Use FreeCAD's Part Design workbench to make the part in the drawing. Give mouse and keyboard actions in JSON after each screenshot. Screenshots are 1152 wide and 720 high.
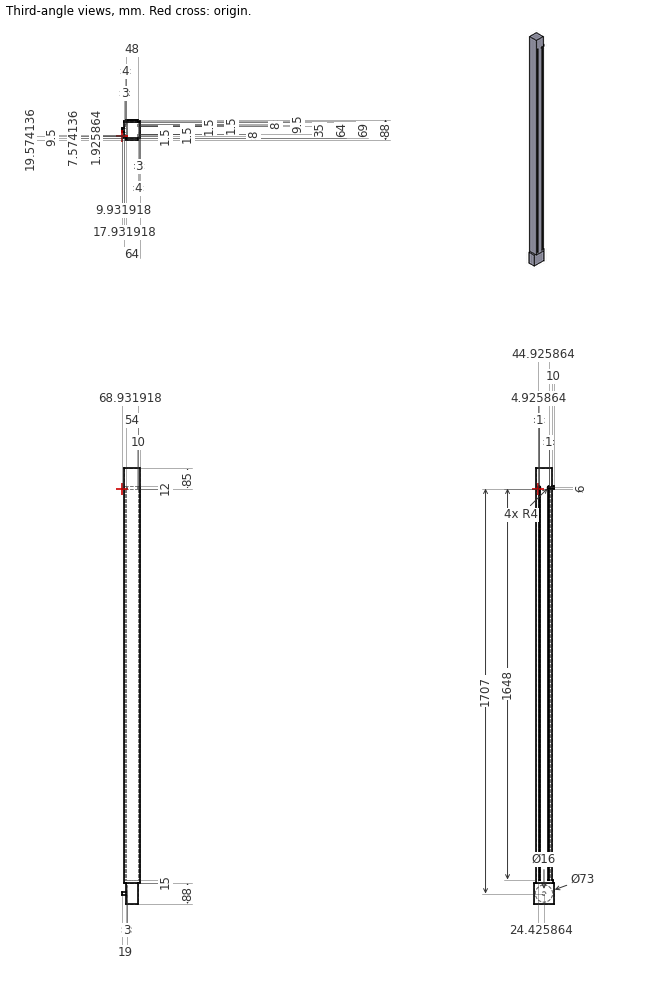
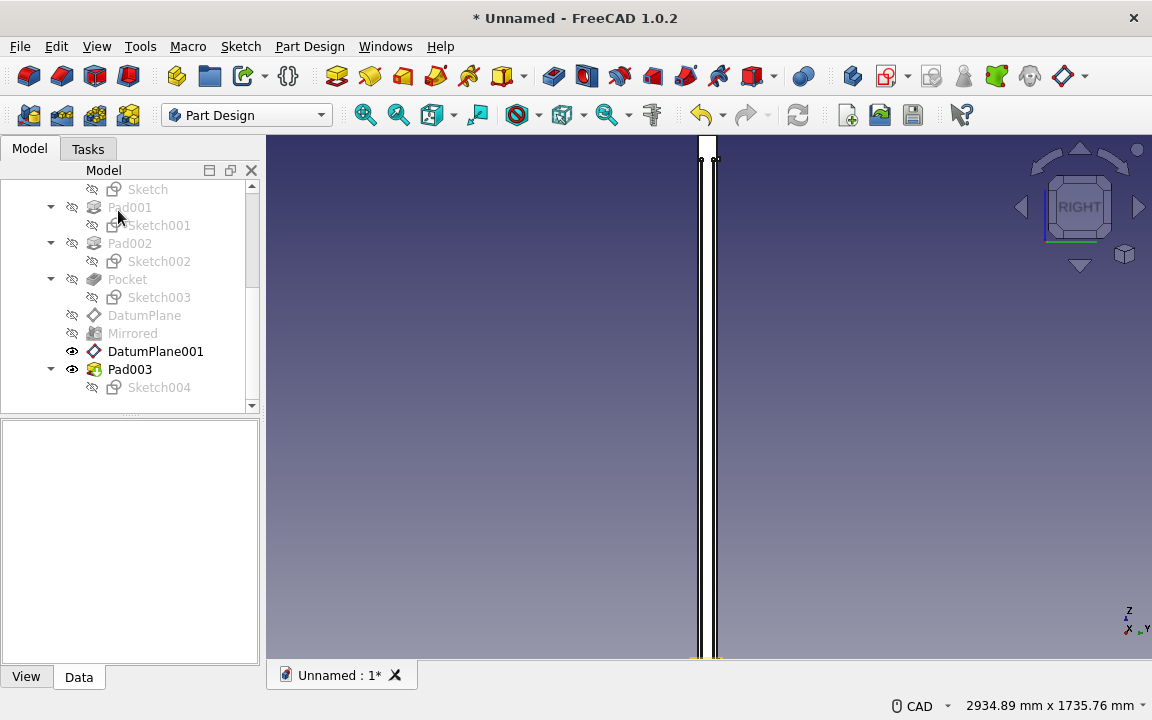
{"action": "left_click", "coordinate": [117, 351]}
{"action": "key", "text": "space"}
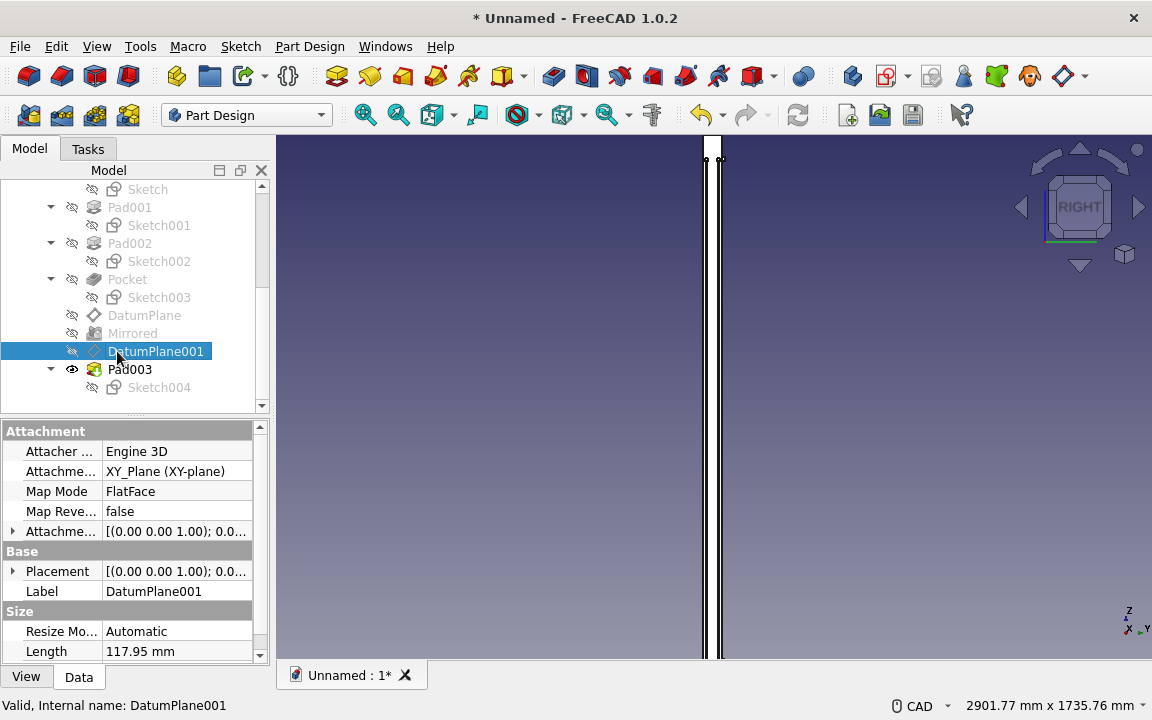
{"action": "left_click", "coordinate": [366, 116]}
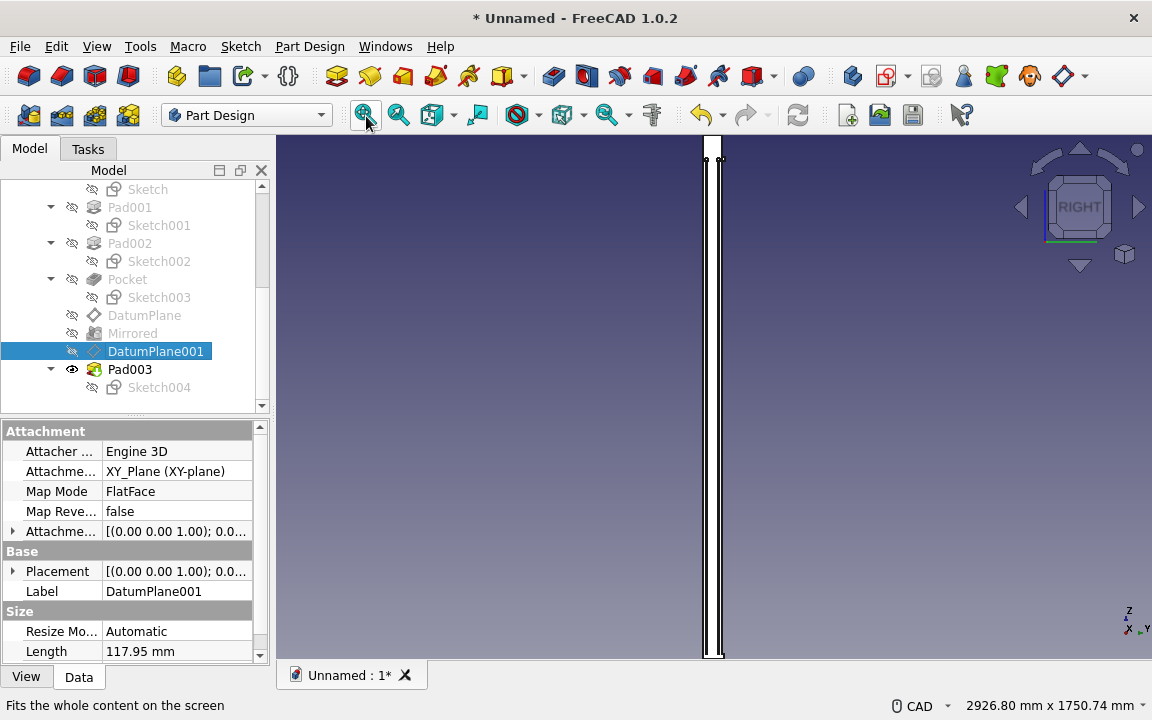
{"action": "key", "text": "5"}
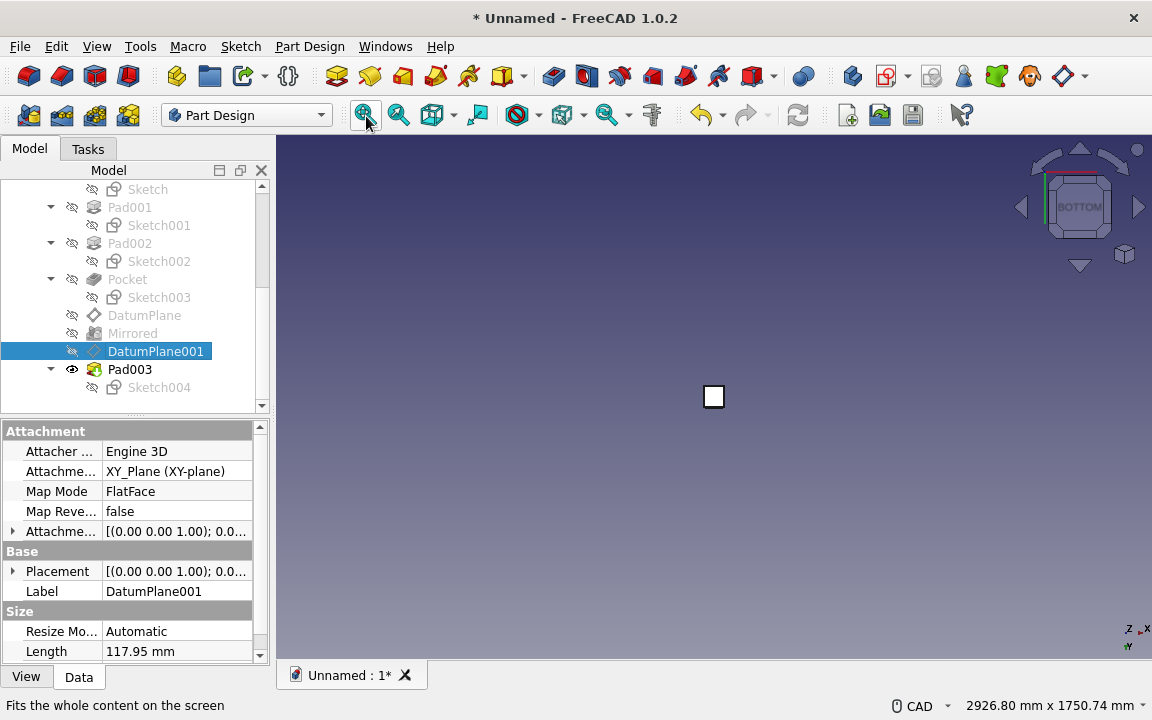
{"action": "left_click", "coordinate": [366, 116]}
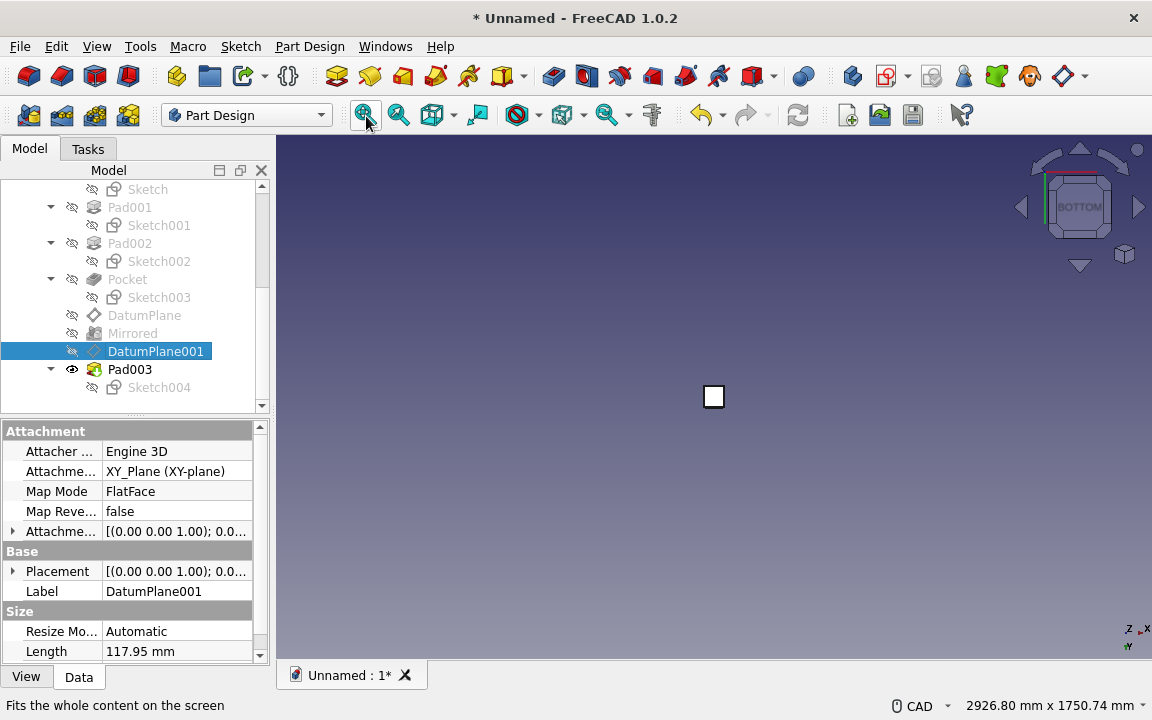
{"action": "left_click", "coordinate": [714, 395]}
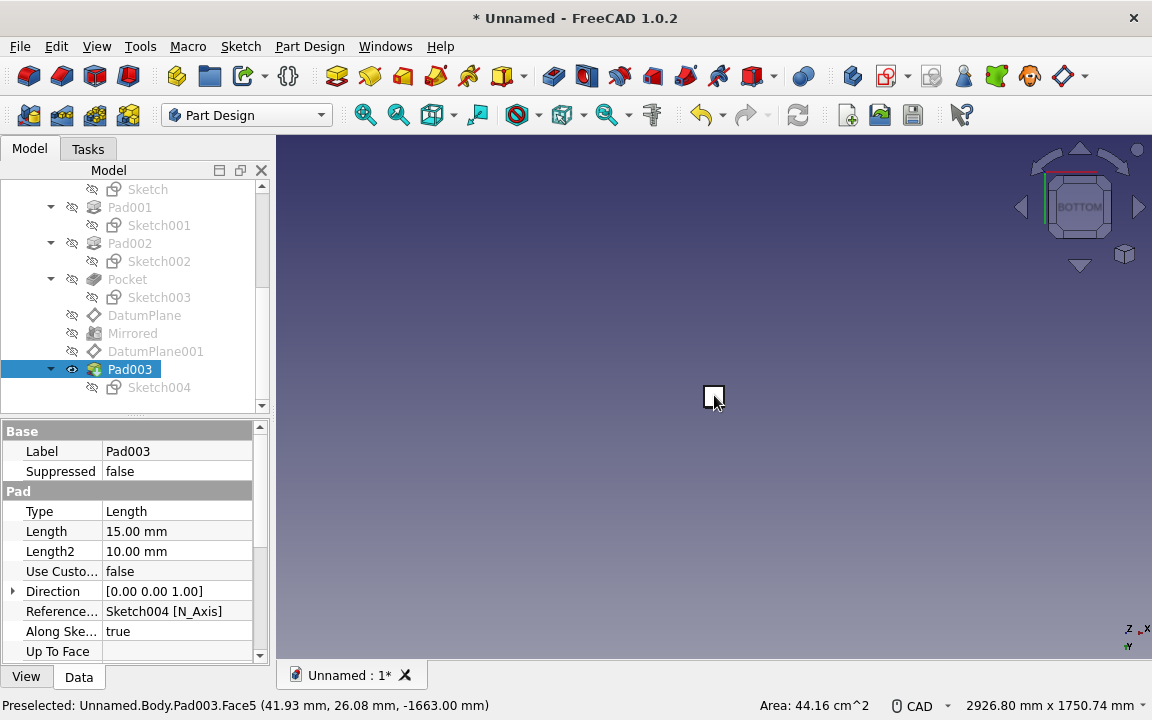
{"action": "left_click", "coordinate": [886, 76]}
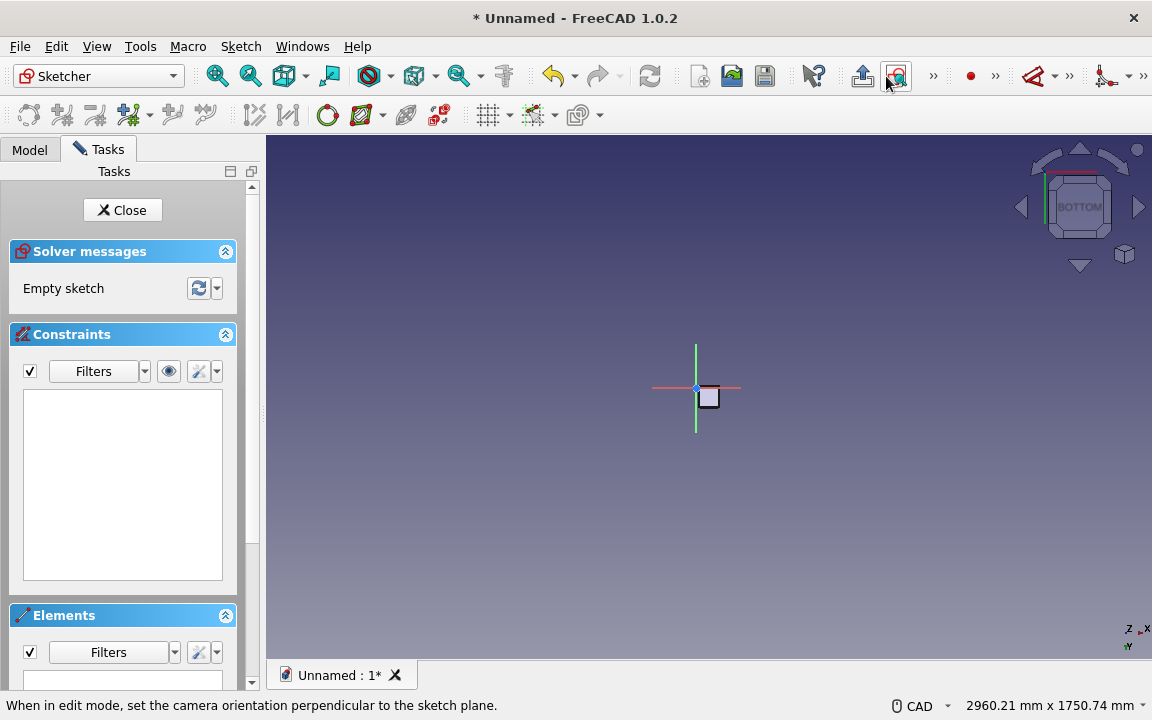
{"action": "scroll", "coordinate": [712, 395], "scroll_direction": "up", "scroll_amount": 13}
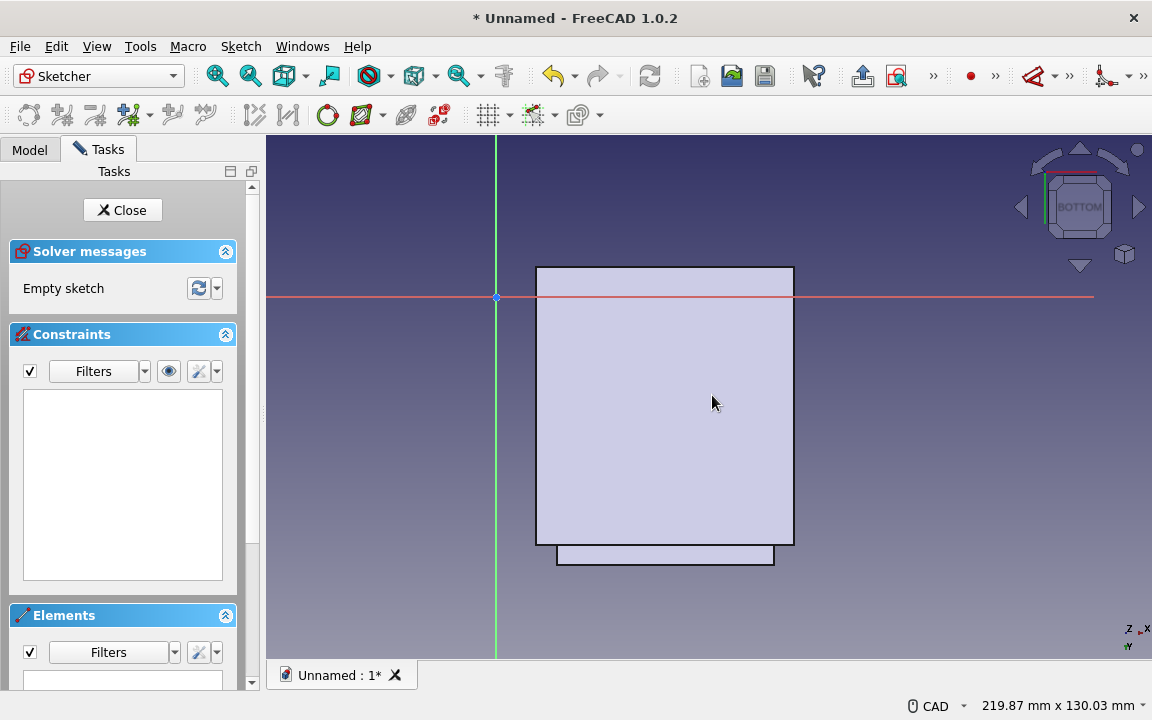
{"action": "key", "text": "g r"}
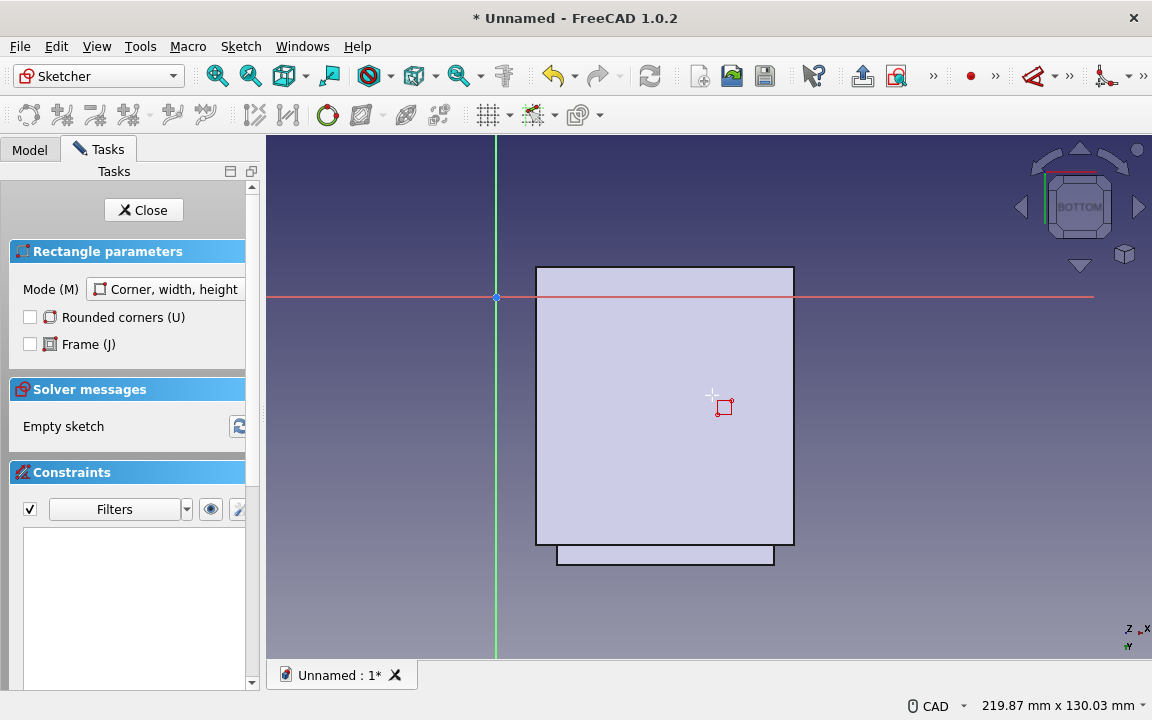
{"action": "left_click", "coordinate": [569, 218]}
{"action": "mouse_move", "coordinate": [762, 573]}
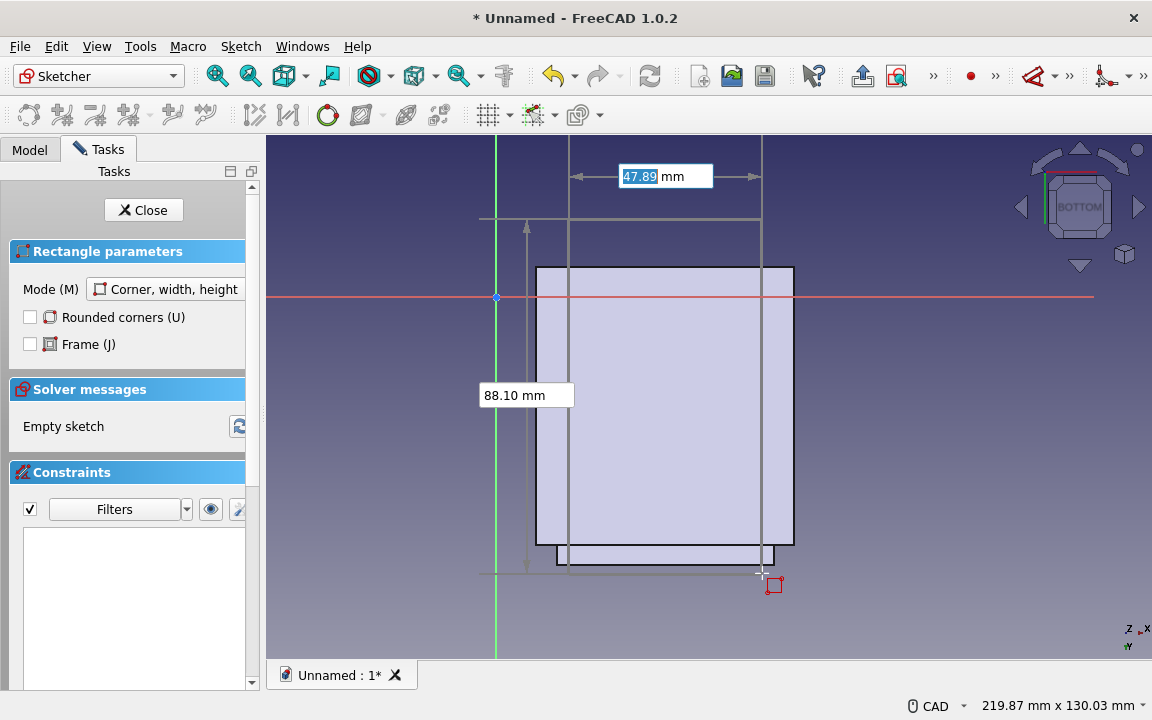
{"action": "type", "text": "48"}
{"action": "key", "text": "Tab"}
{"action": "type", "text": "88"}
{"action": "key", "text": "Return"}
{"action": "key", "text": "Escape"}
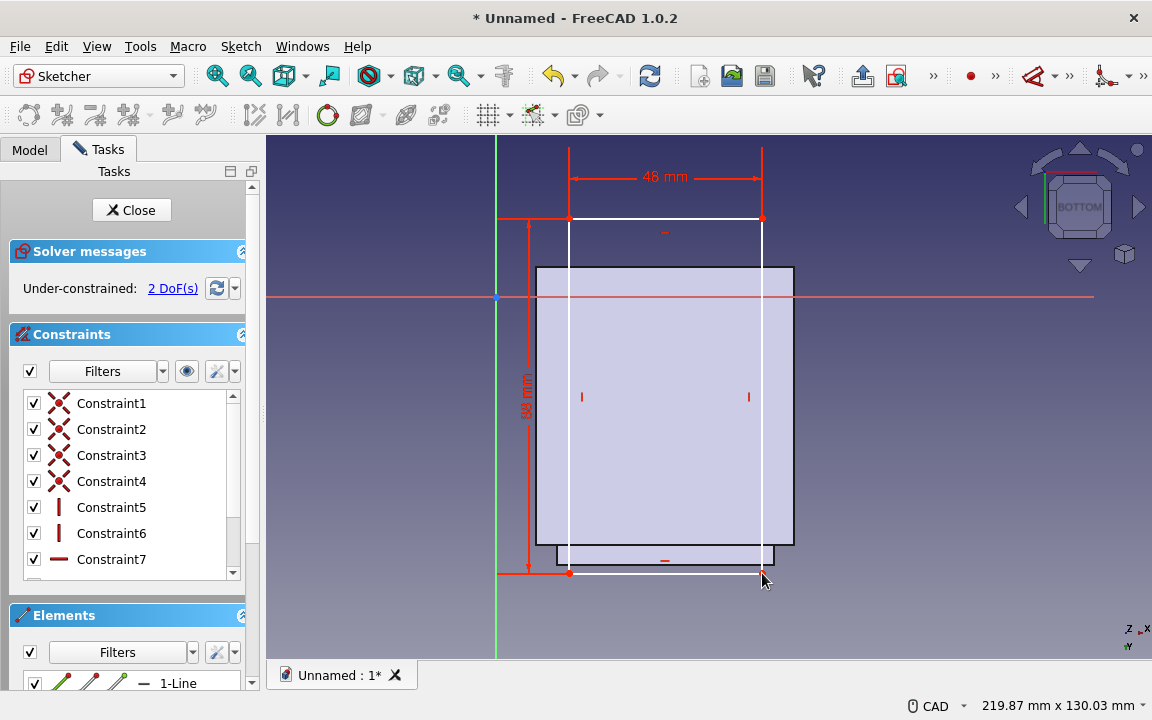
{"action": "left_click", "coordinate": [1032, 76]}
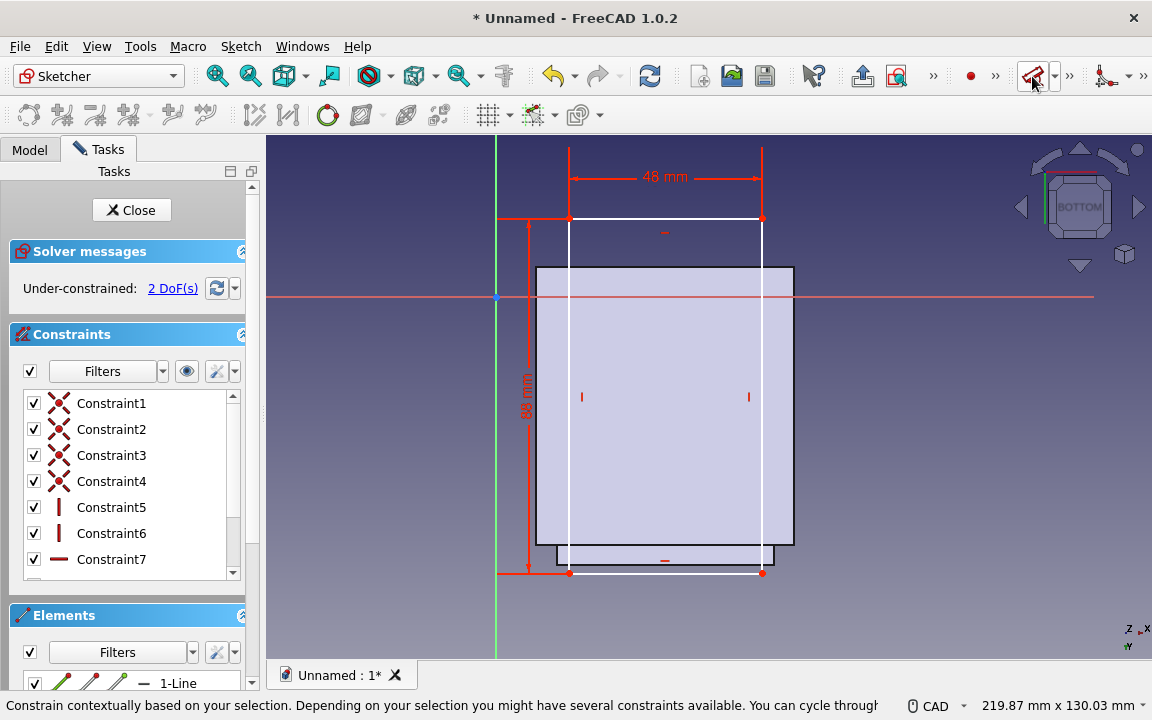
{"action": "left_click", "coordinate": [569, 219]}
{"action": "left_click", "coordinate": [533, 185]}